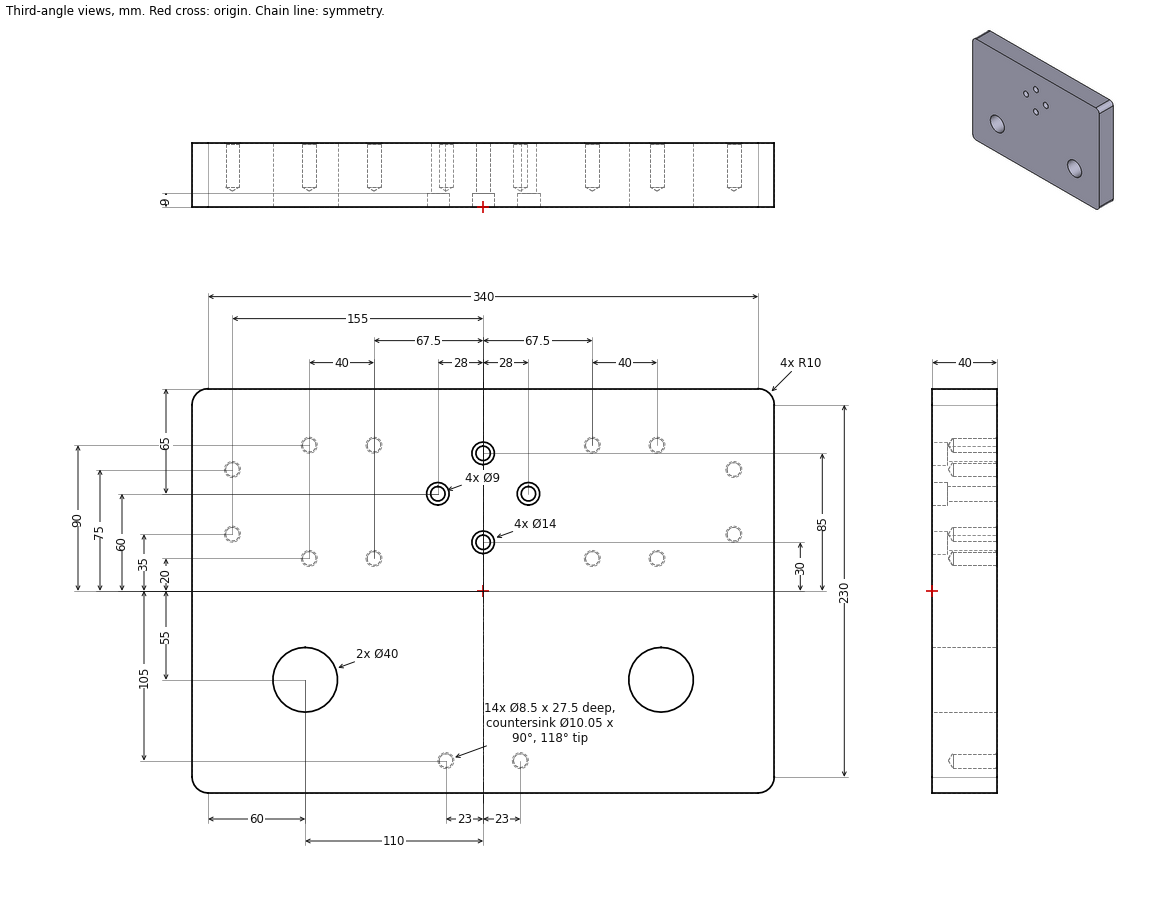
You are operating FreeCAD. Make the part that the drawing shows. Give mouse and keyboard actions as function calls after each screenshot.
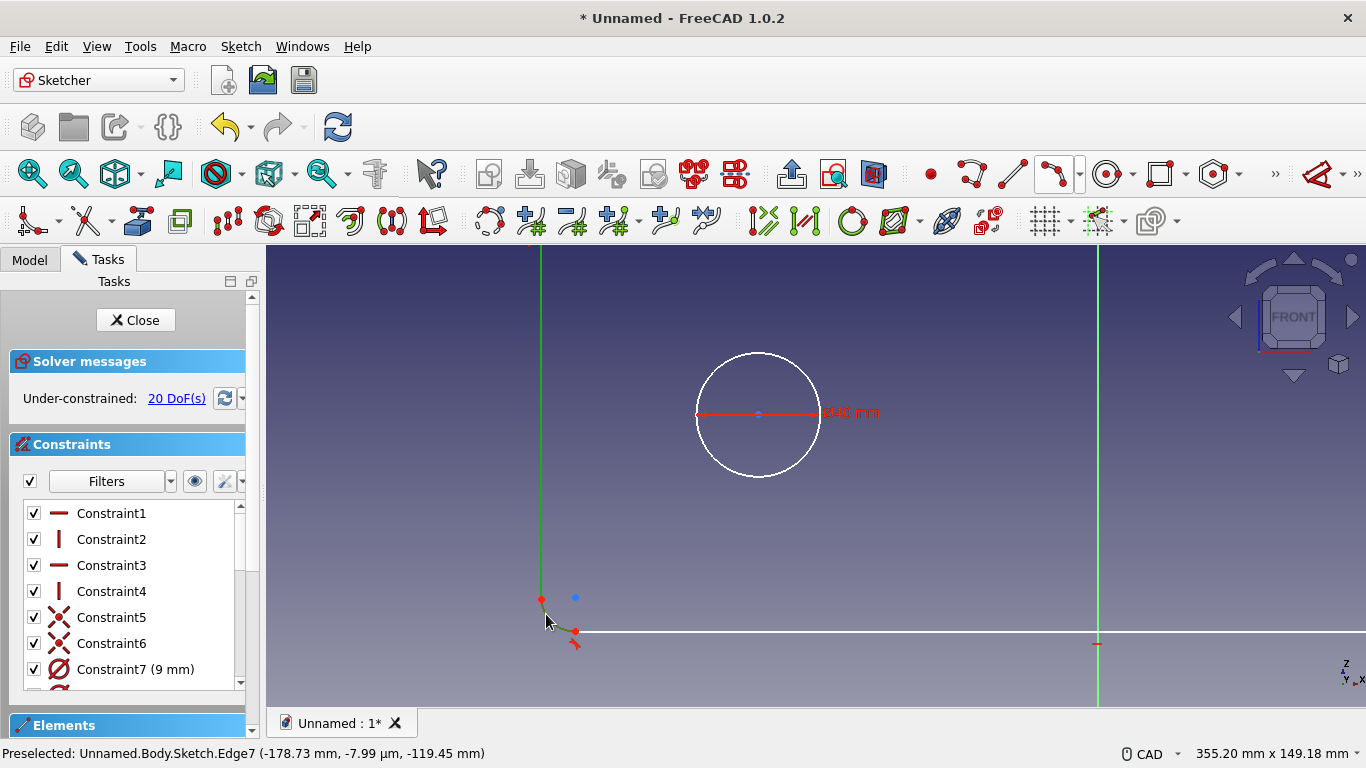
key(t)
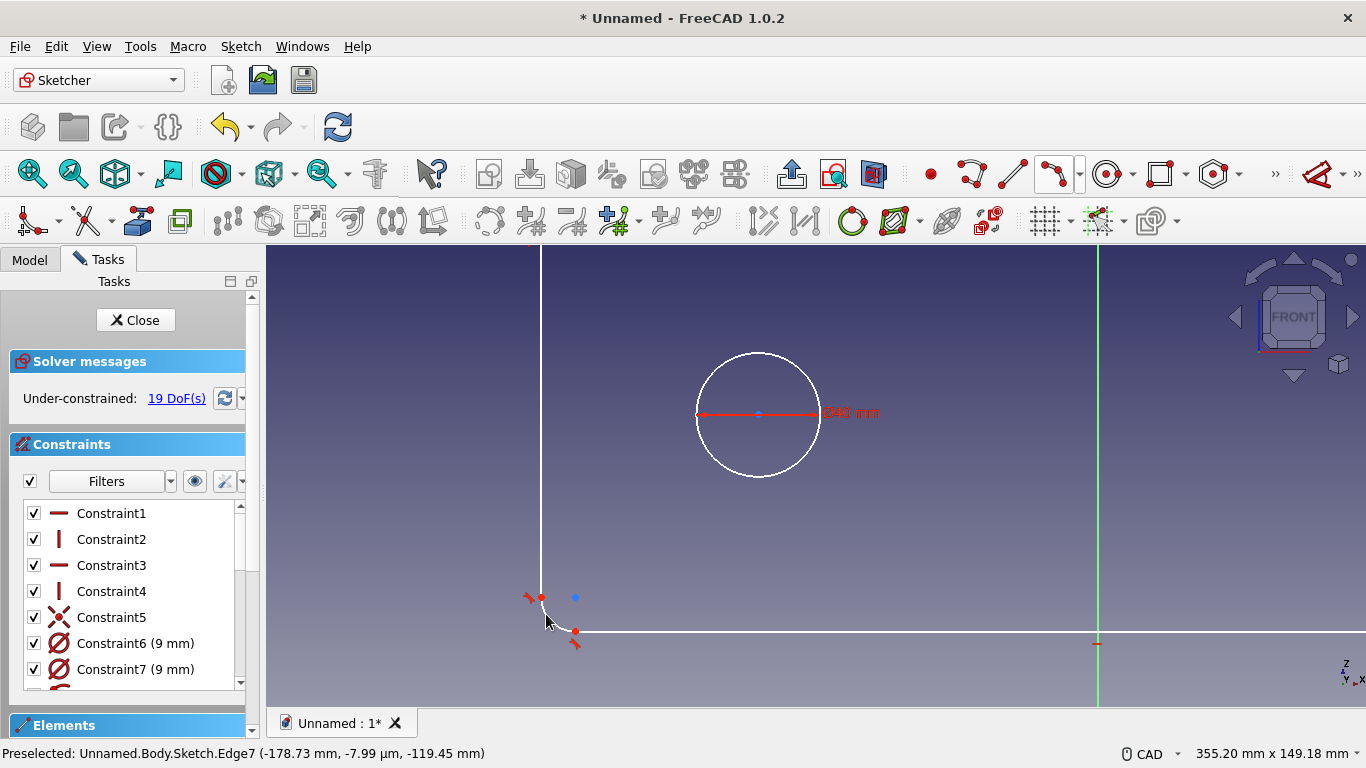
click(541, 384)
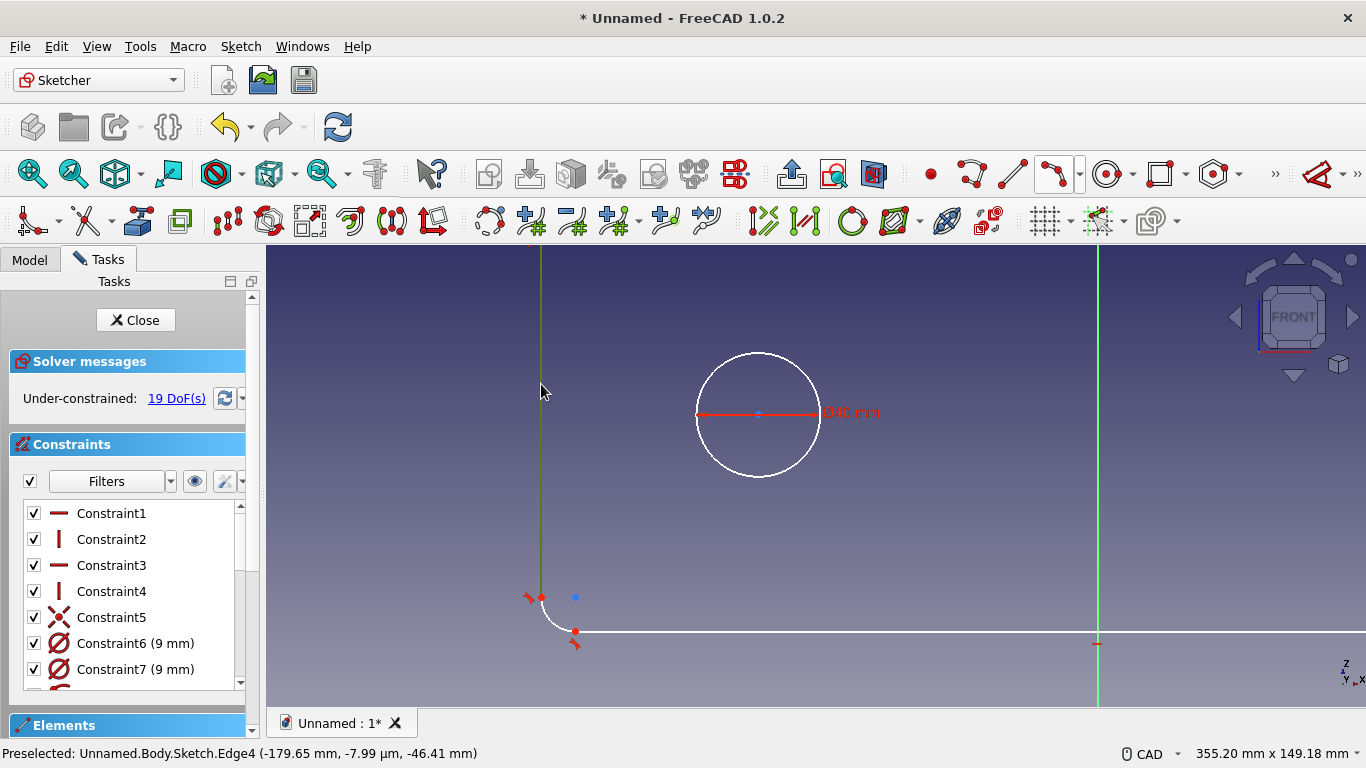
scroll(544, 613, down, 5)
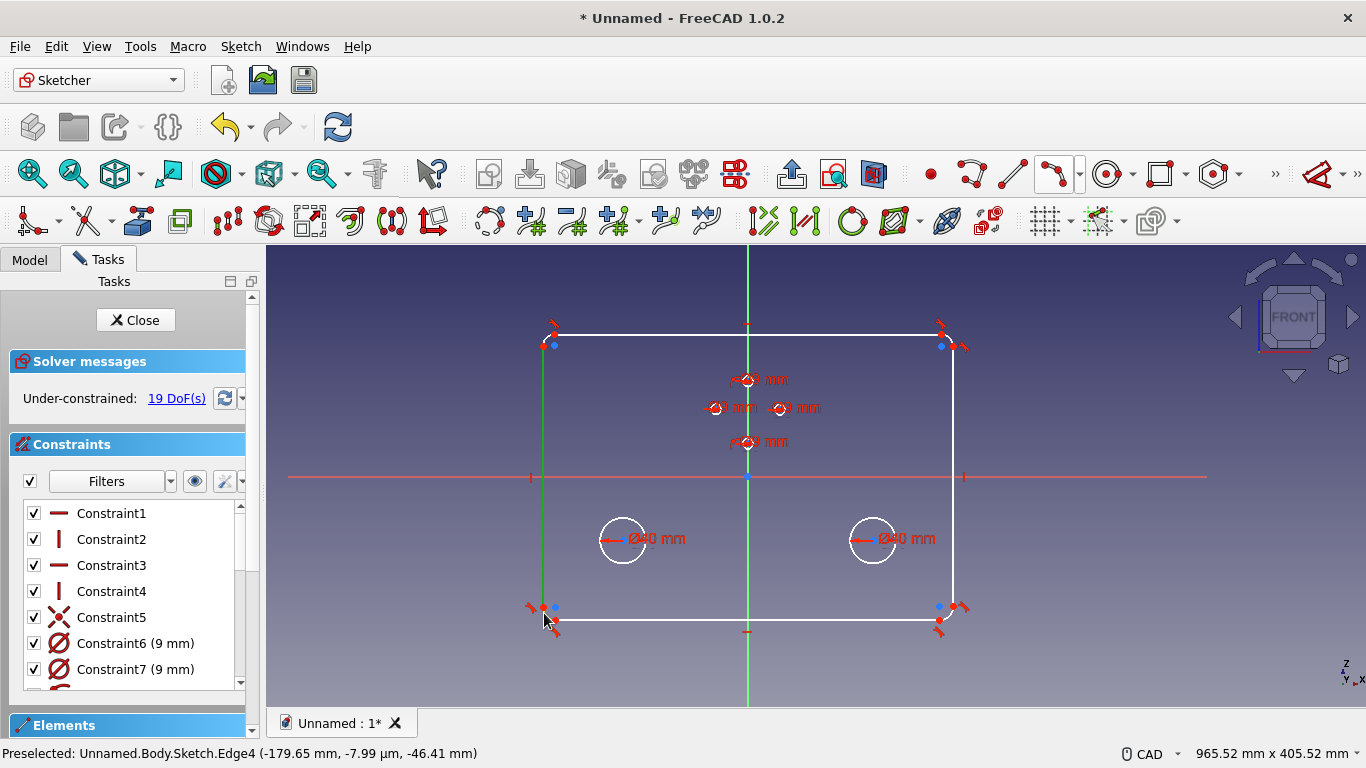
scroll(549, 336, up, 5)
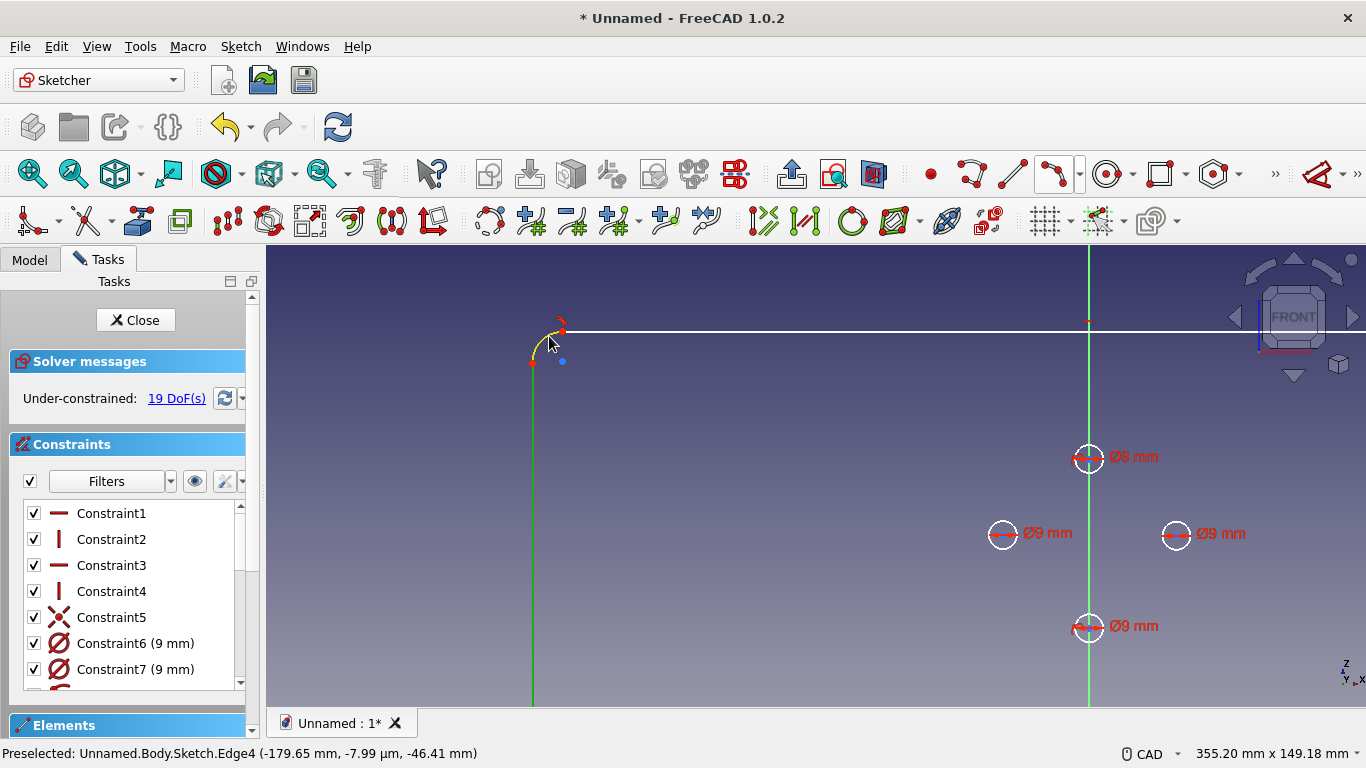
click(548, 335)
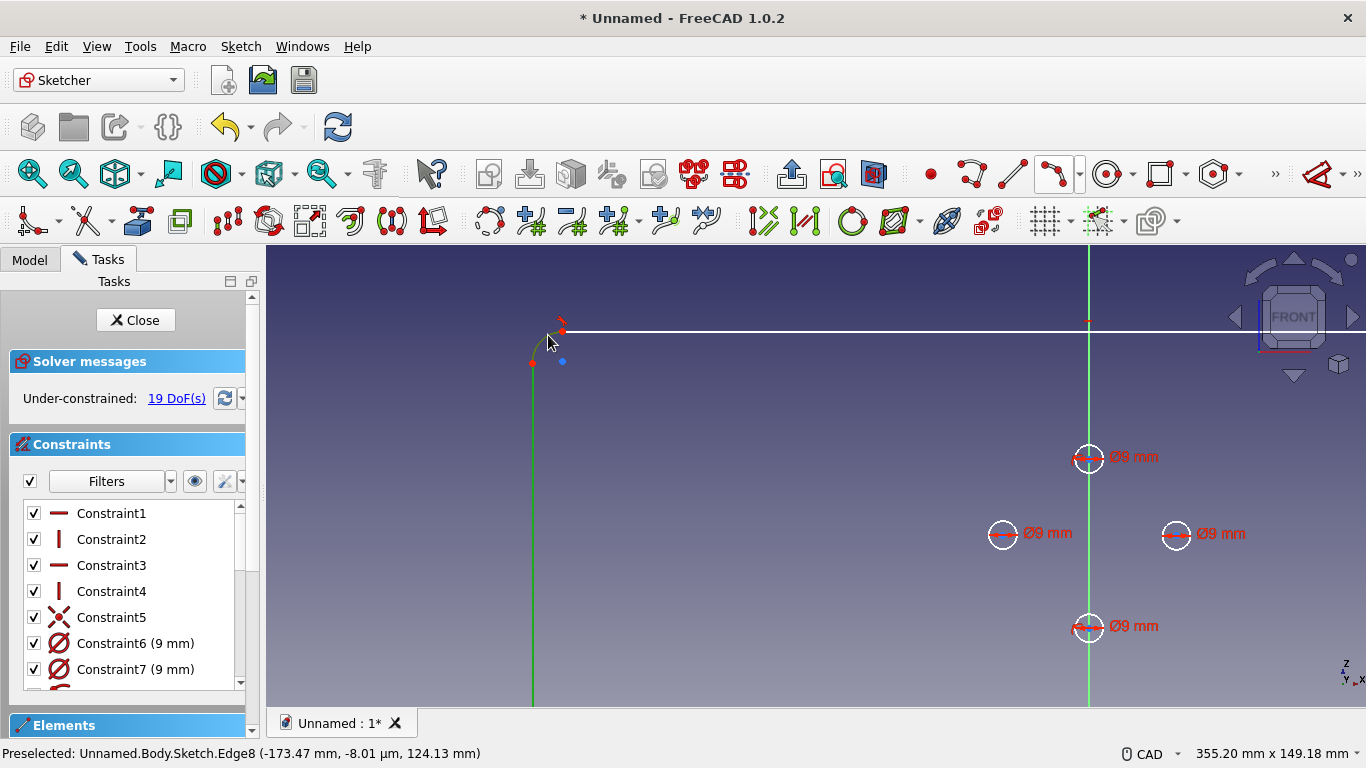
key(t)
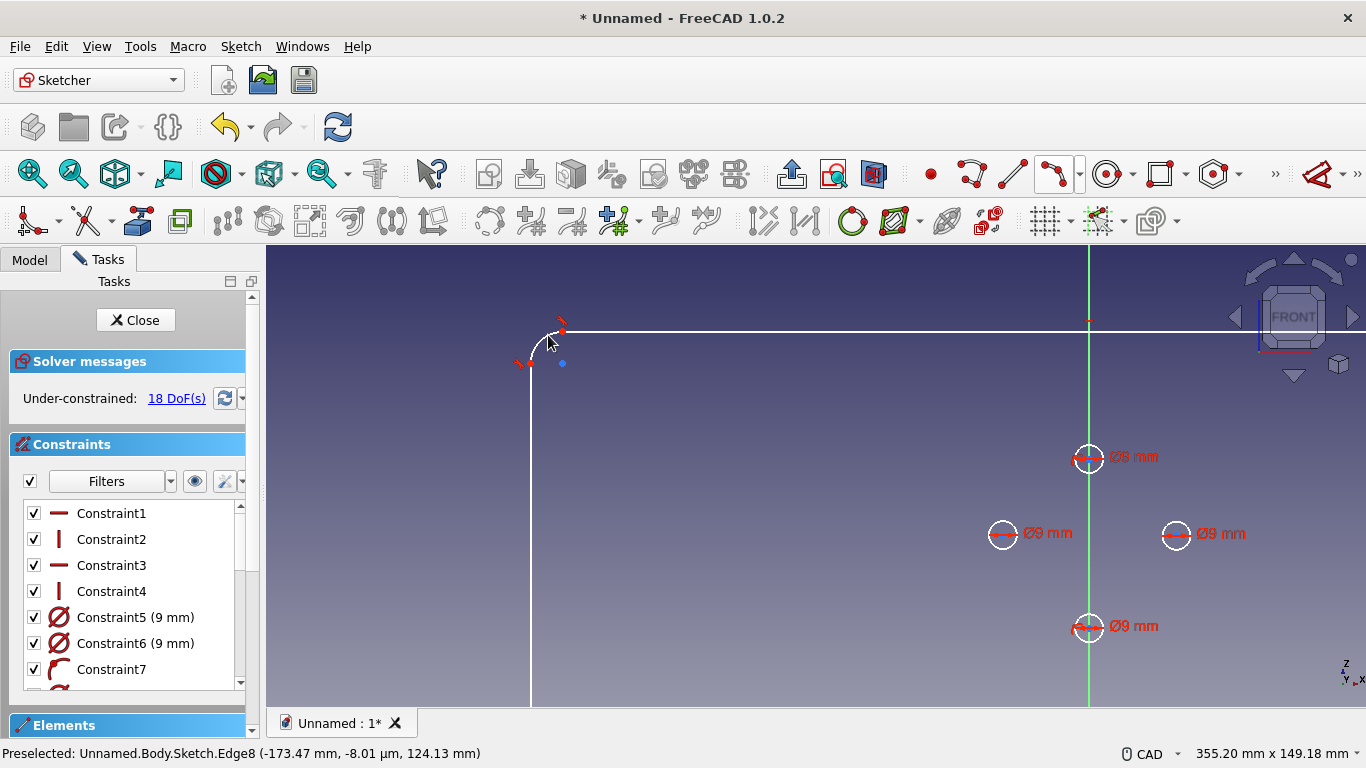
scroll(549, 335, down, 5)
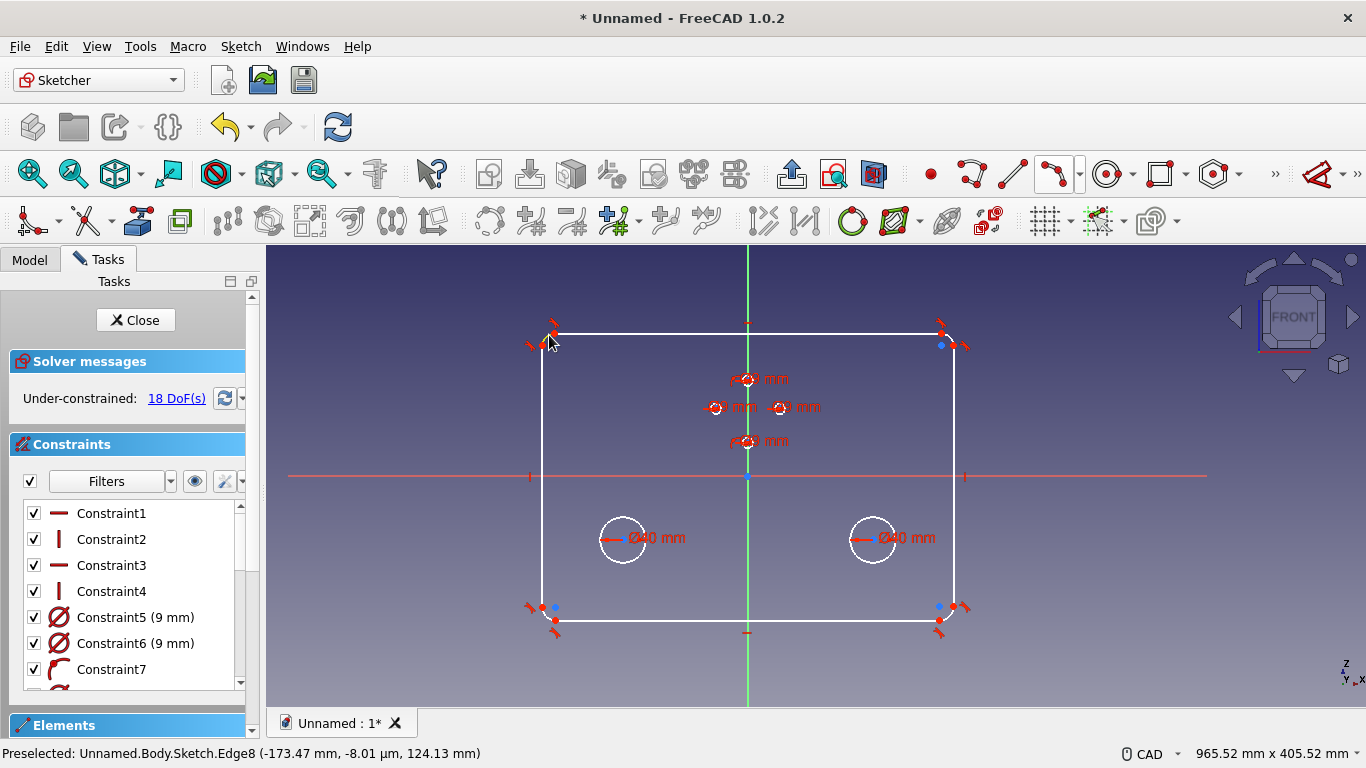
scroll(952, 341, up, 5)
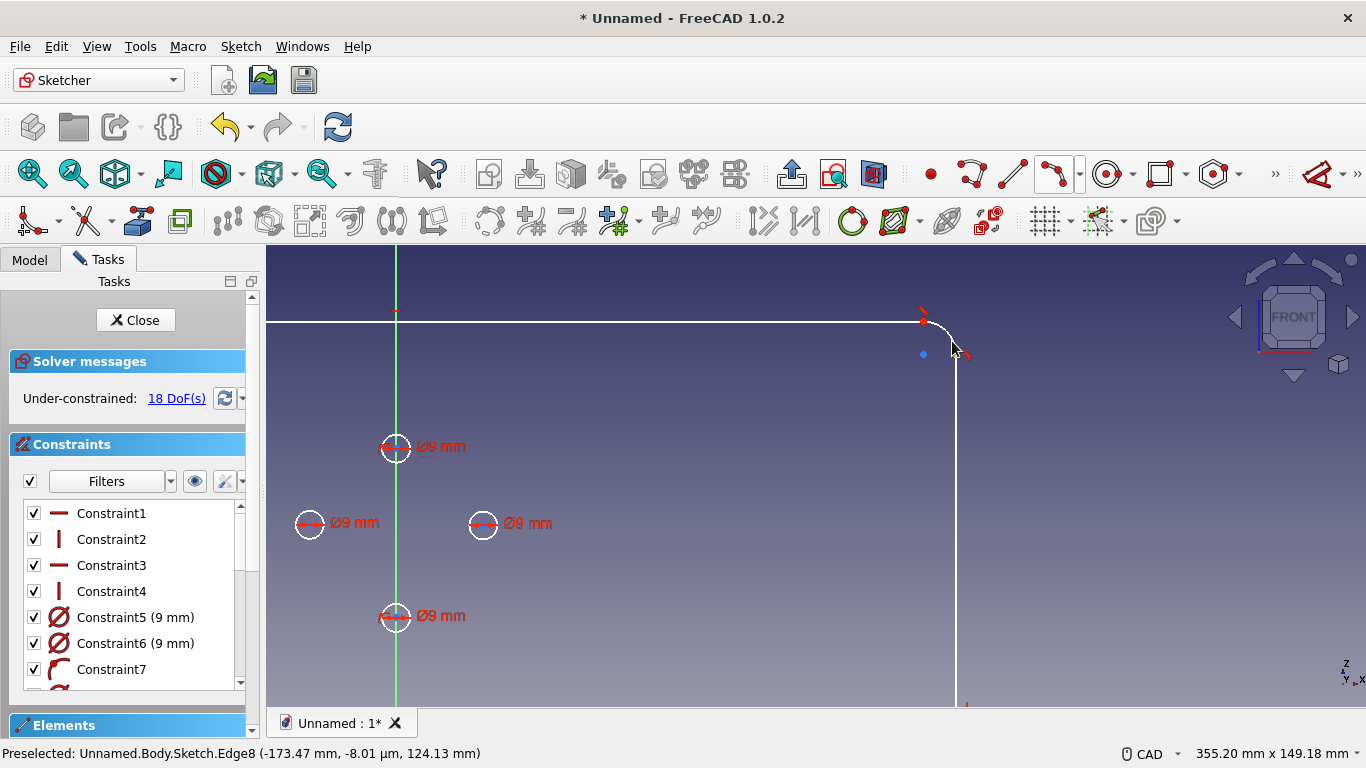
click(952, 339)